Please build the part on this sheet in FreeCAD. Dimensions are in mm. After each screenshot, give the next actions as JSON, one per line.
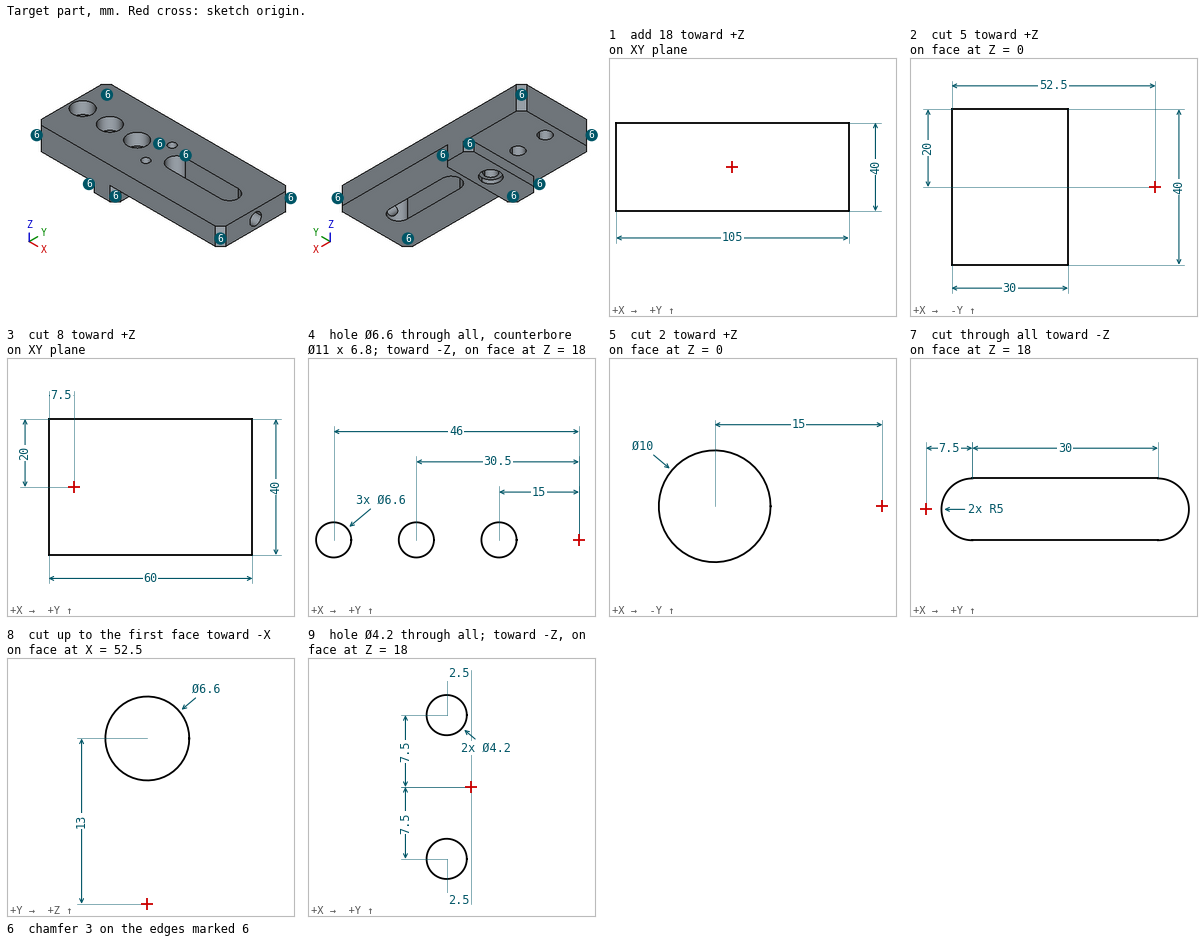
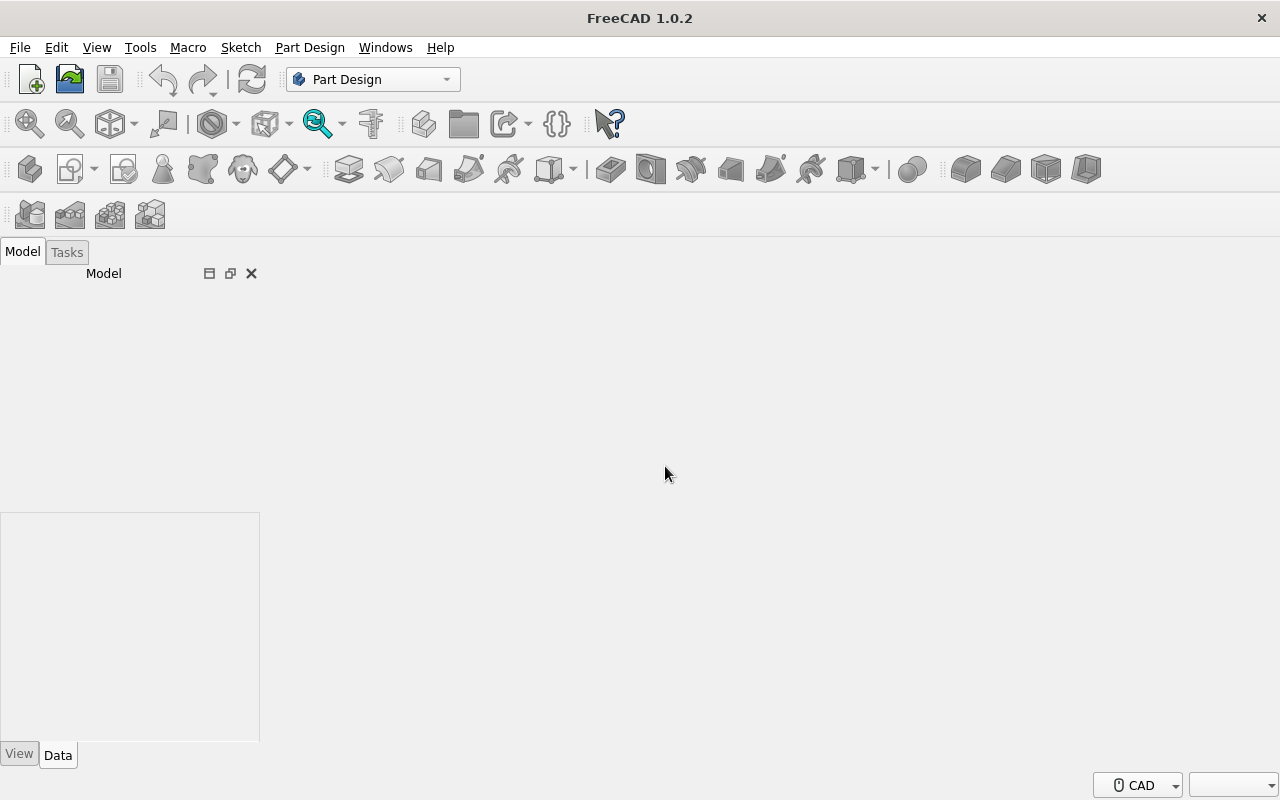
{"action": "key", "text": "ctrl+n"}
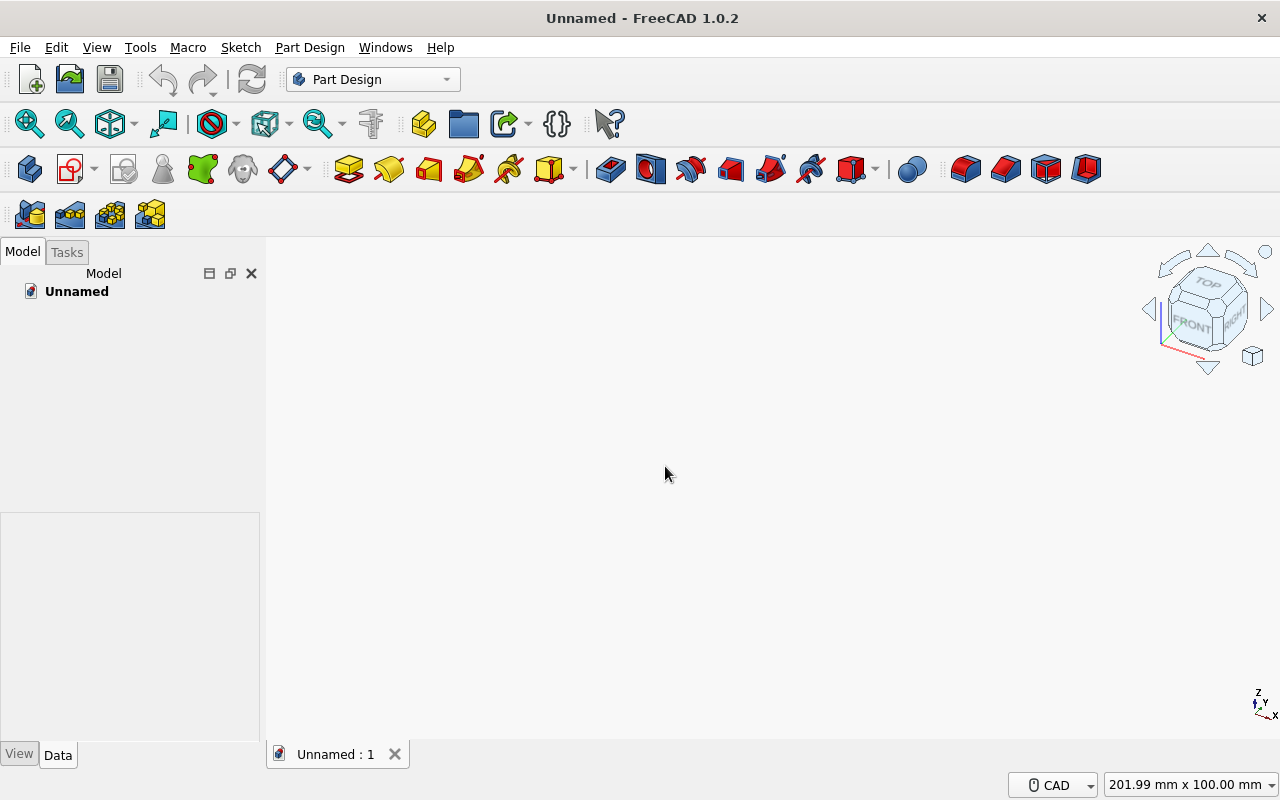
{"action": "left_click", "coordinate": [70, 170]}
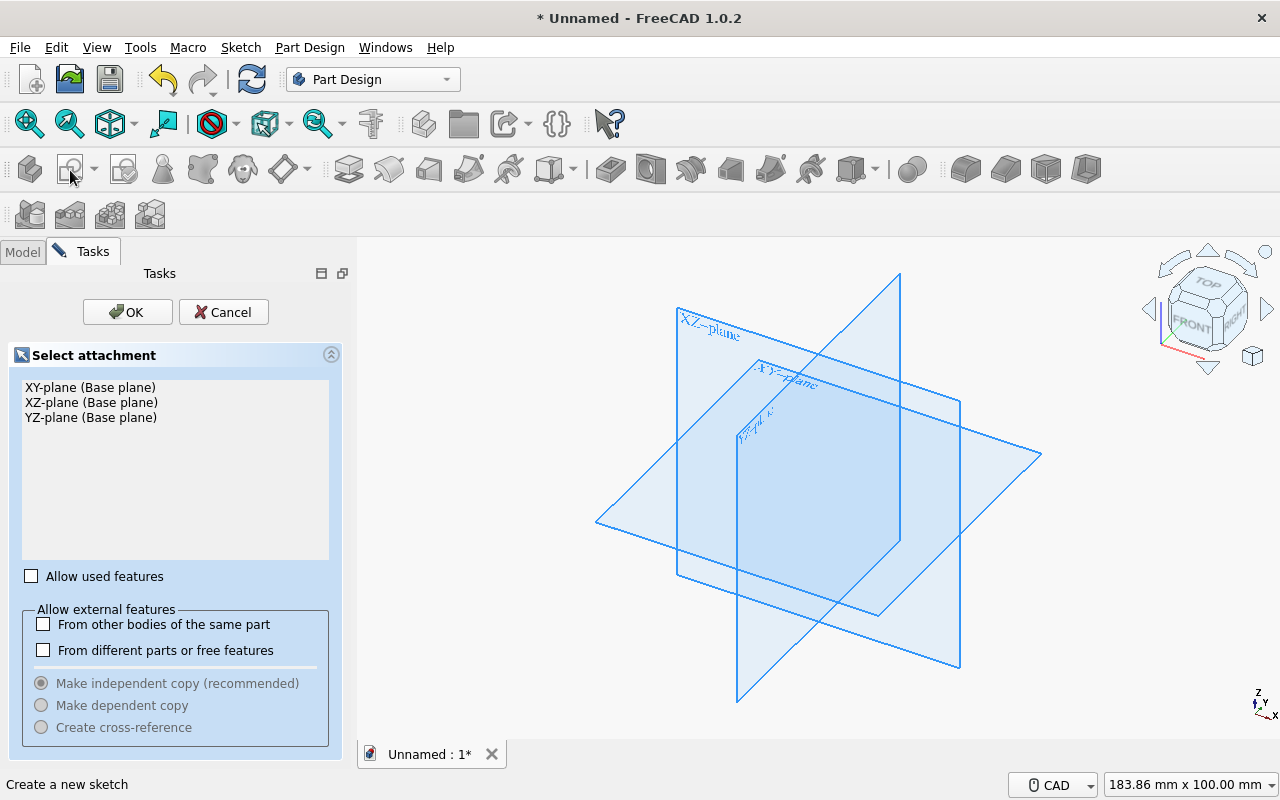
{"action": "left_click", "coordinate": [82, 388]}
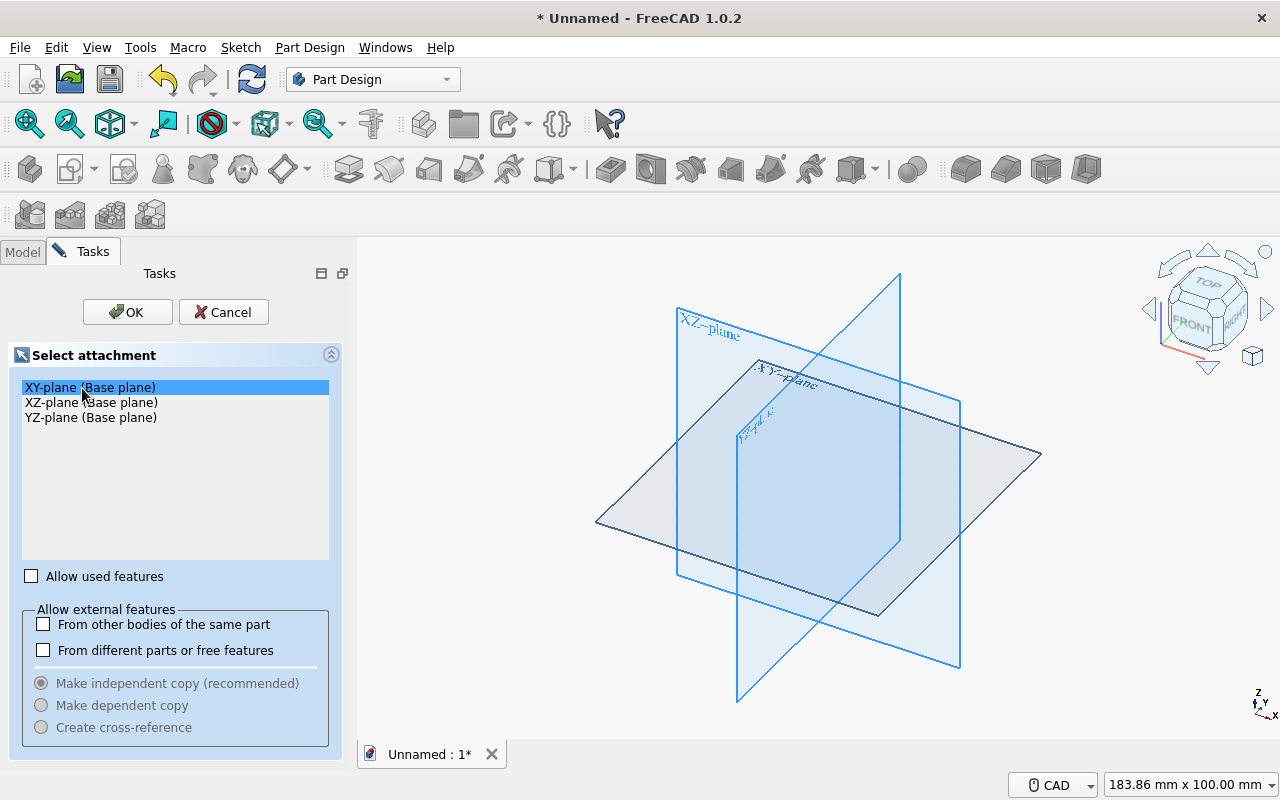
{"action": "left_click", "coordinate": [128, 312]}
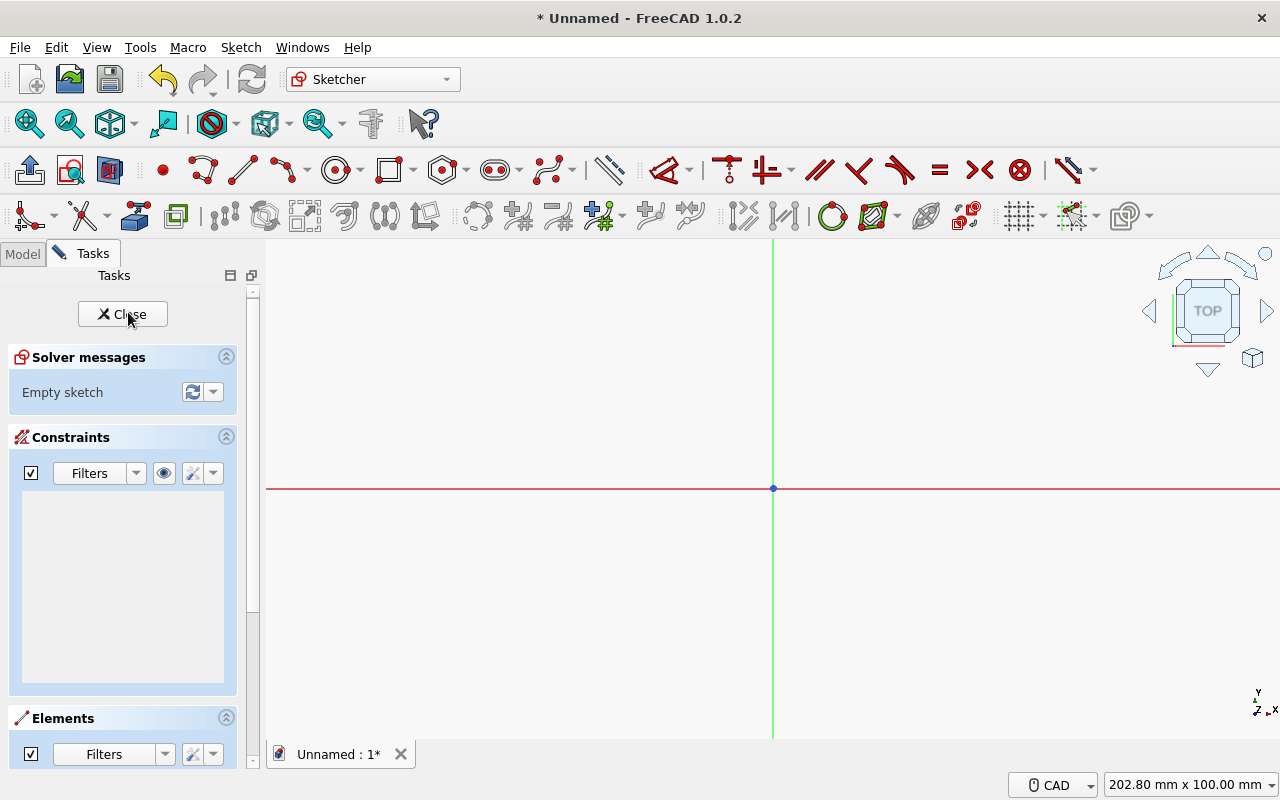
{"action": "left_click", "coordinate": [416, 170]}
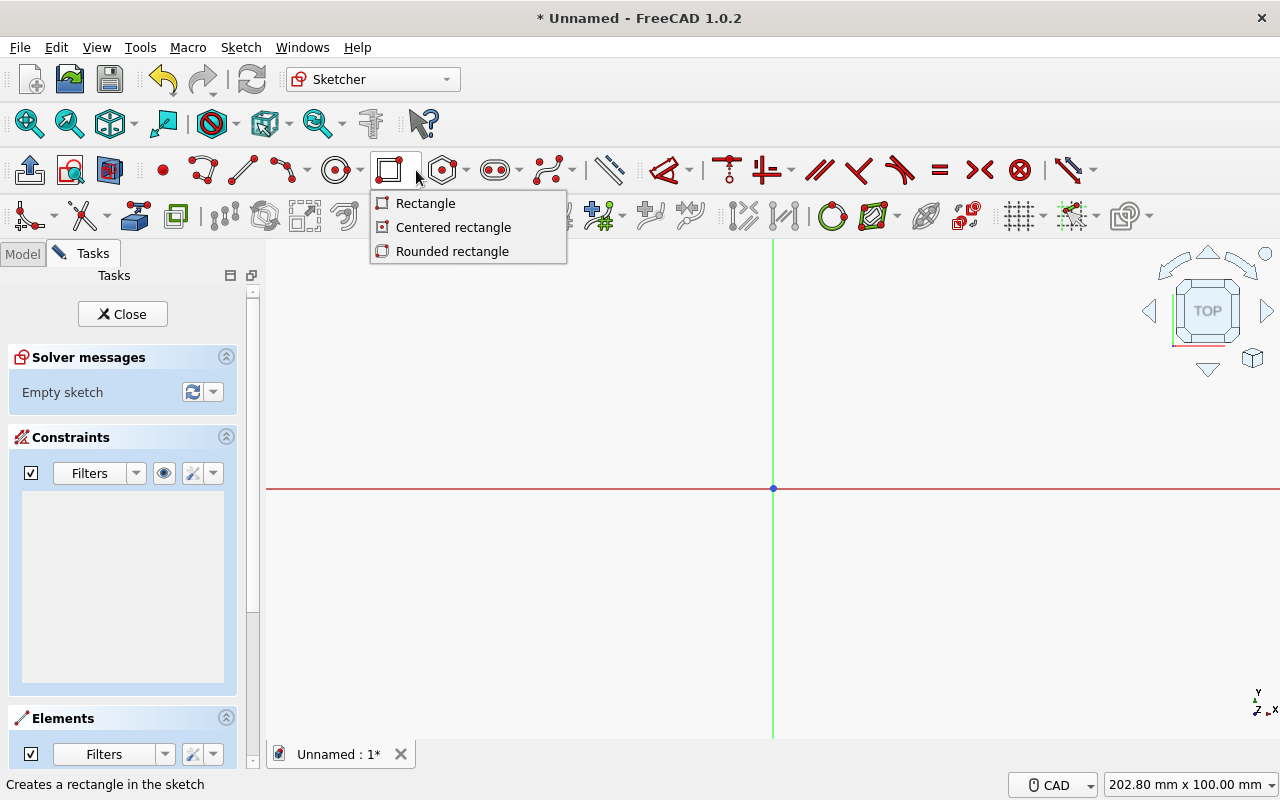
{"action": "left_click", "coordinate": [468, 227]}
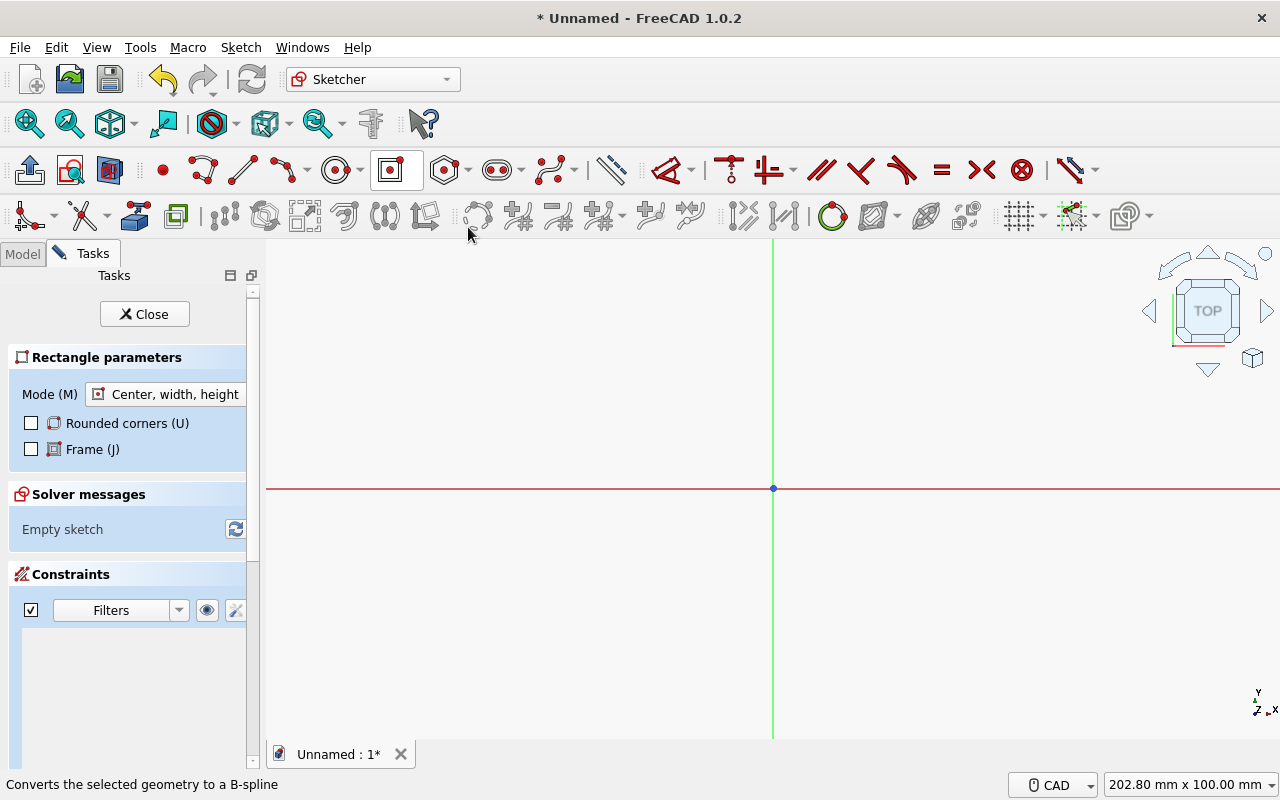
{"action": "left_click", "coordinate": [773, 489]}
{"action": "mouse_move", "coordinate": [1036, 389]}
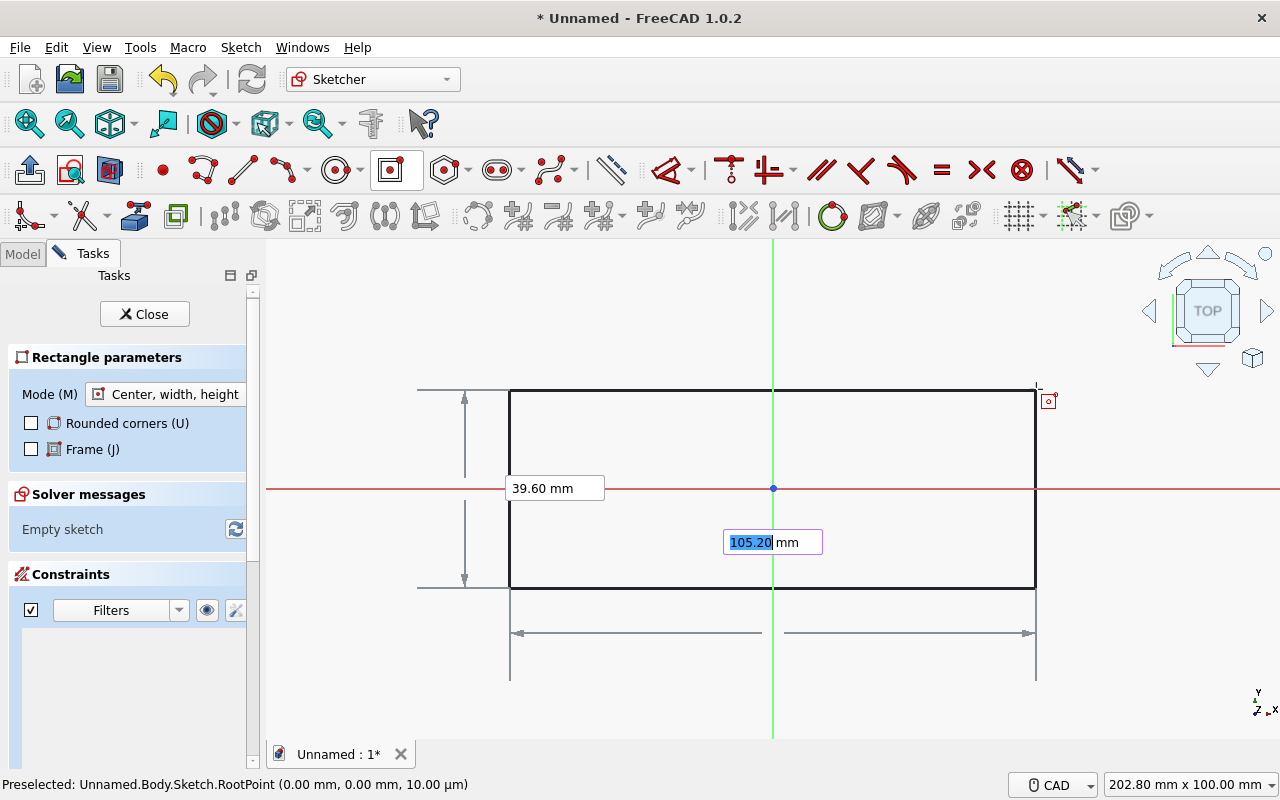
{"action": "type", "text": "105"}
{"action": "key", "text": "Tab"}
{"action": "type", "text": "40"}
{"action": "key", "text": "Return"}
{"action": "key", "text": "Escape"}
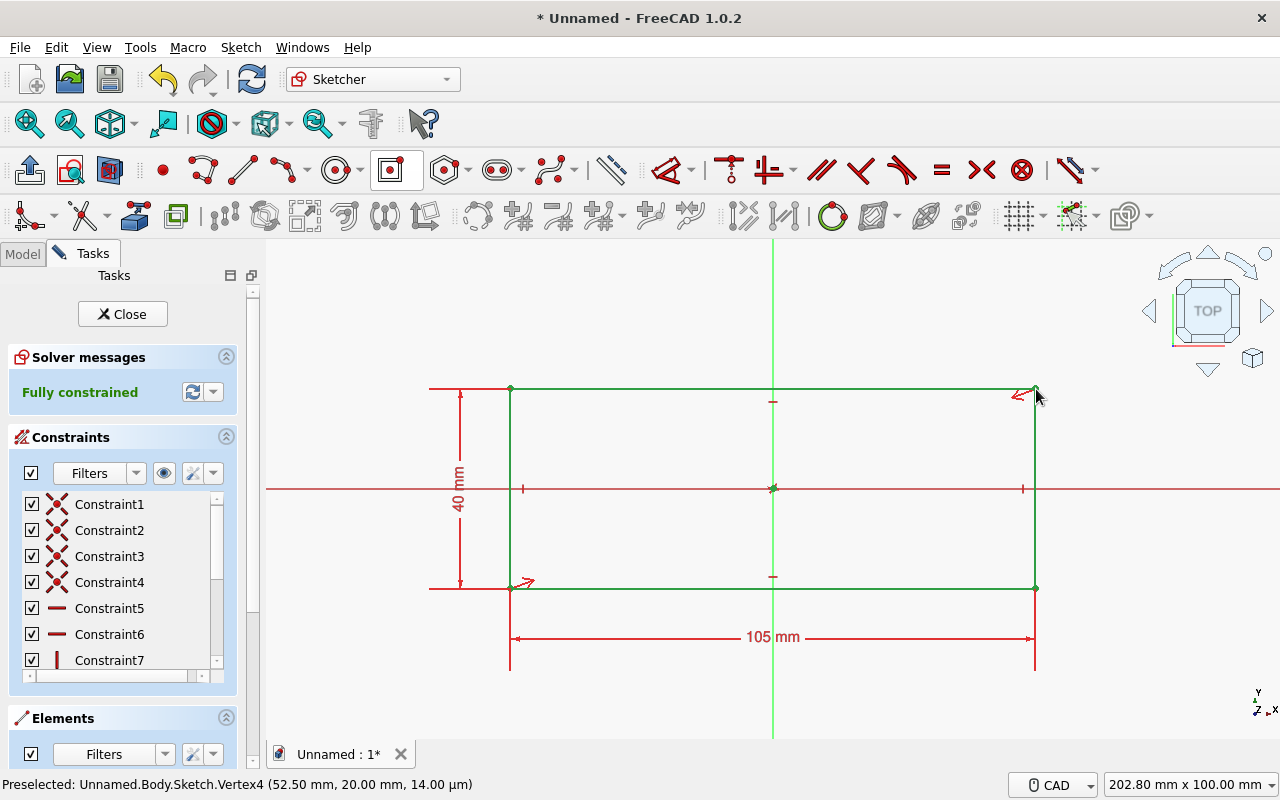
{"action": "left_click", "coordinate": [123, 314]}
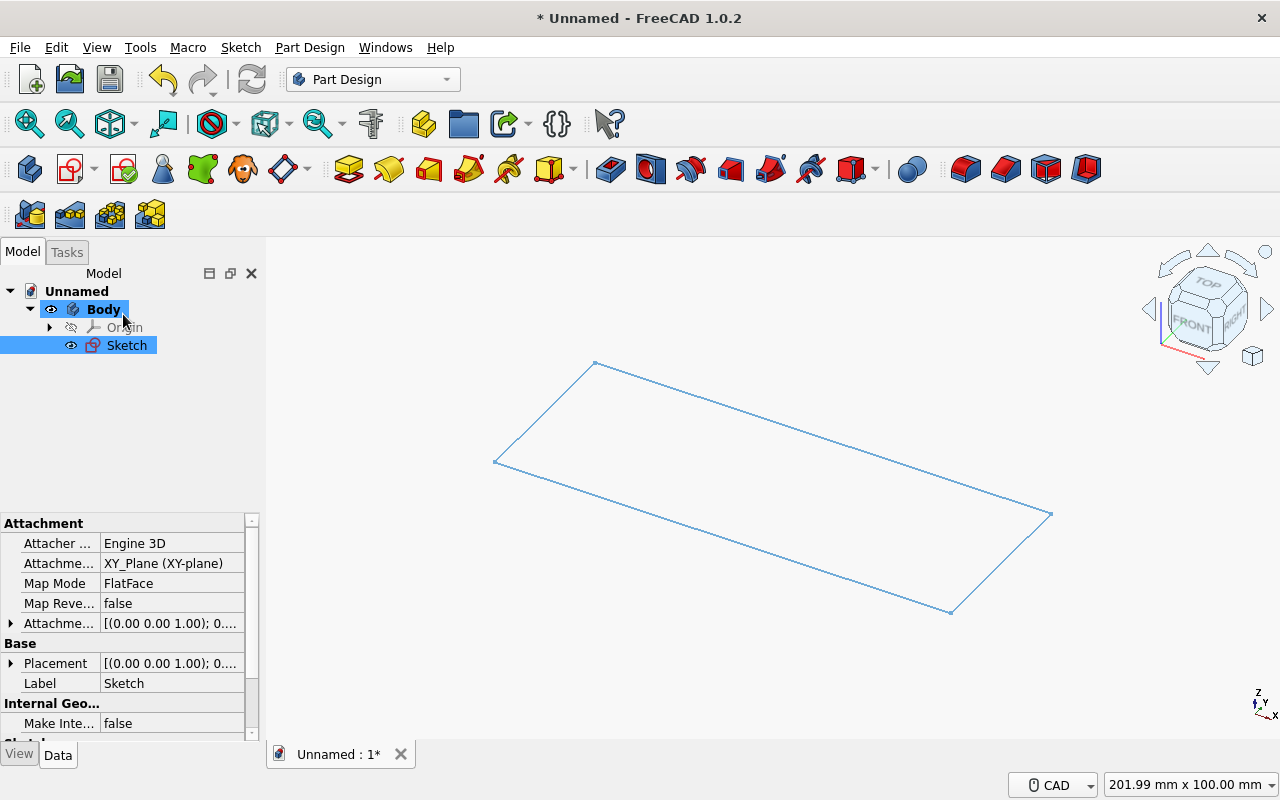
{"action": "left_click", "coordinate": [350, 170]}